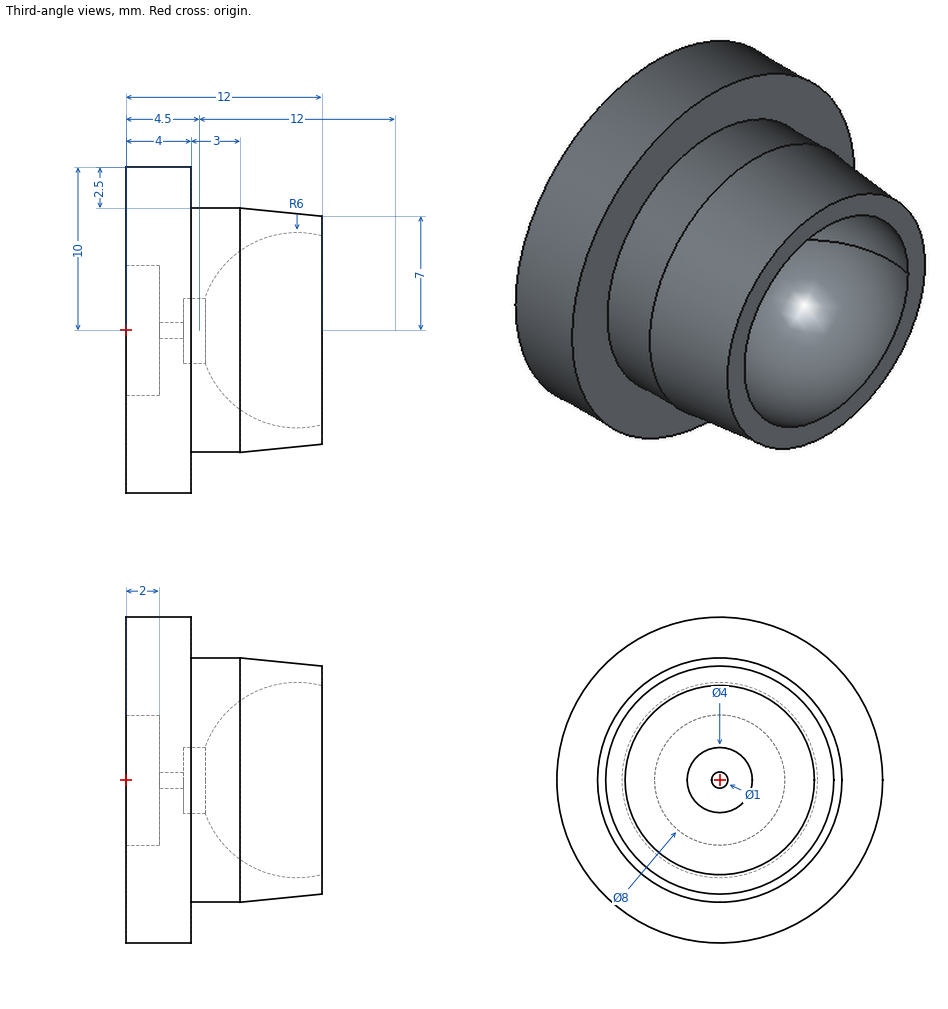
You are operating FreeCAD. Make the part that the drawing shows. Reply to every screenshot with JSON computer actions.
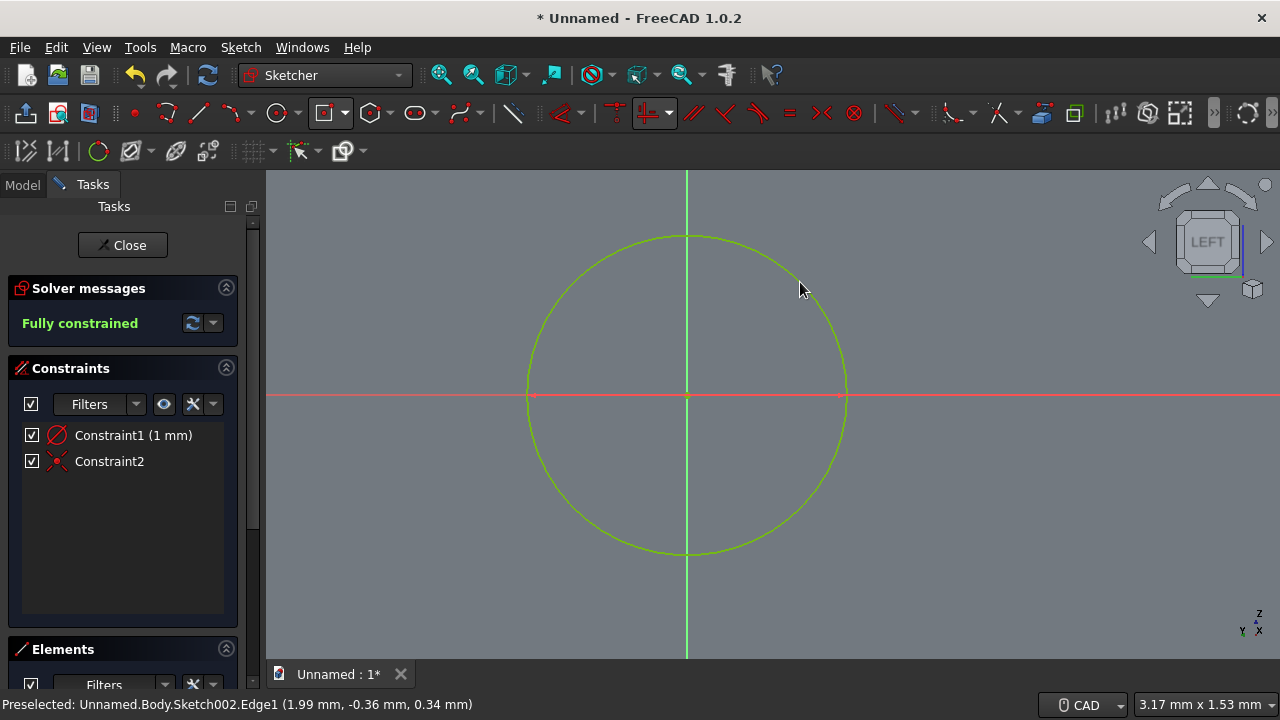
{"action": "left_click", "coordinate": [123, 245]}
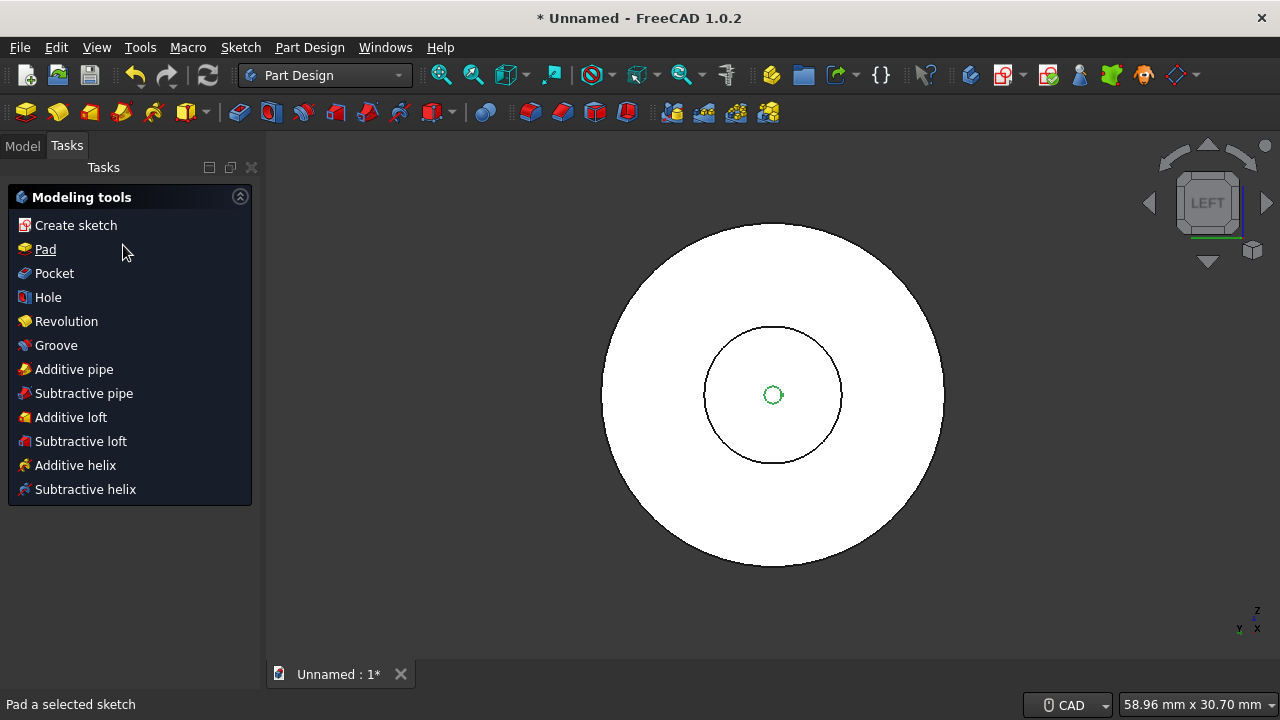
{"action": "left_click", "coordinate": [240, 112]}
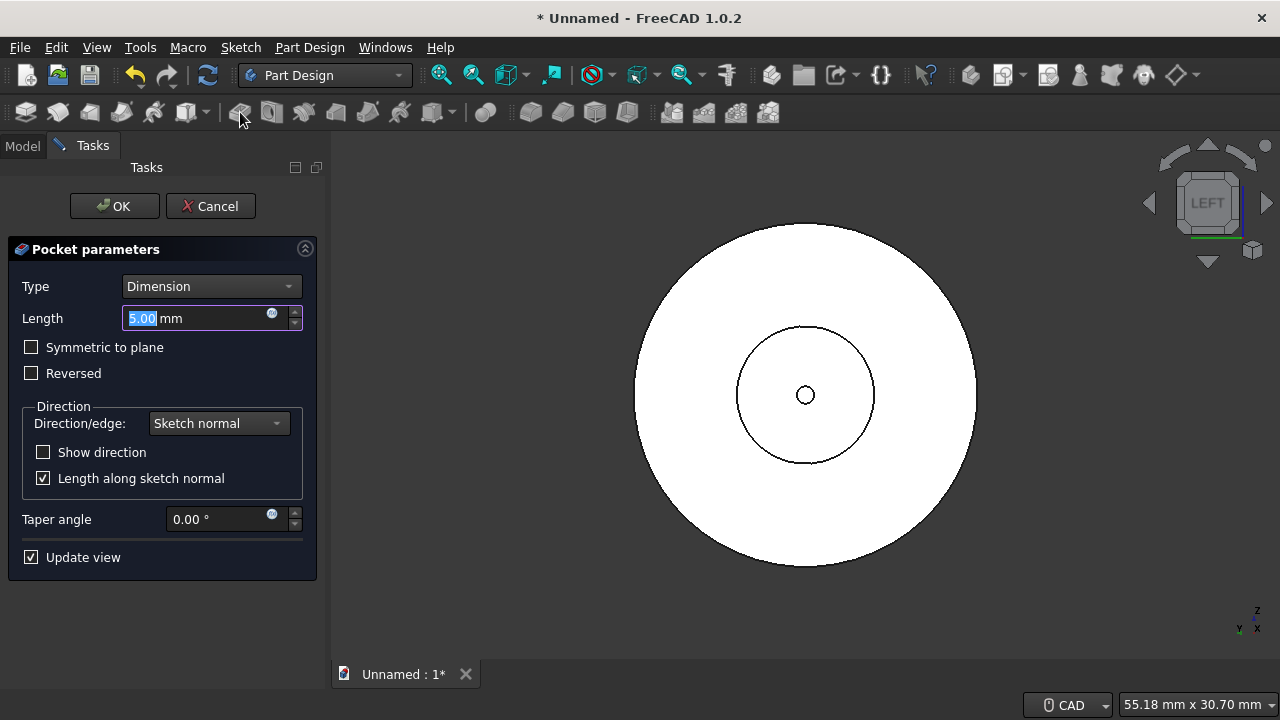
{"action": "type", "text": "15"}
{"action": "key", "text": "Tab"}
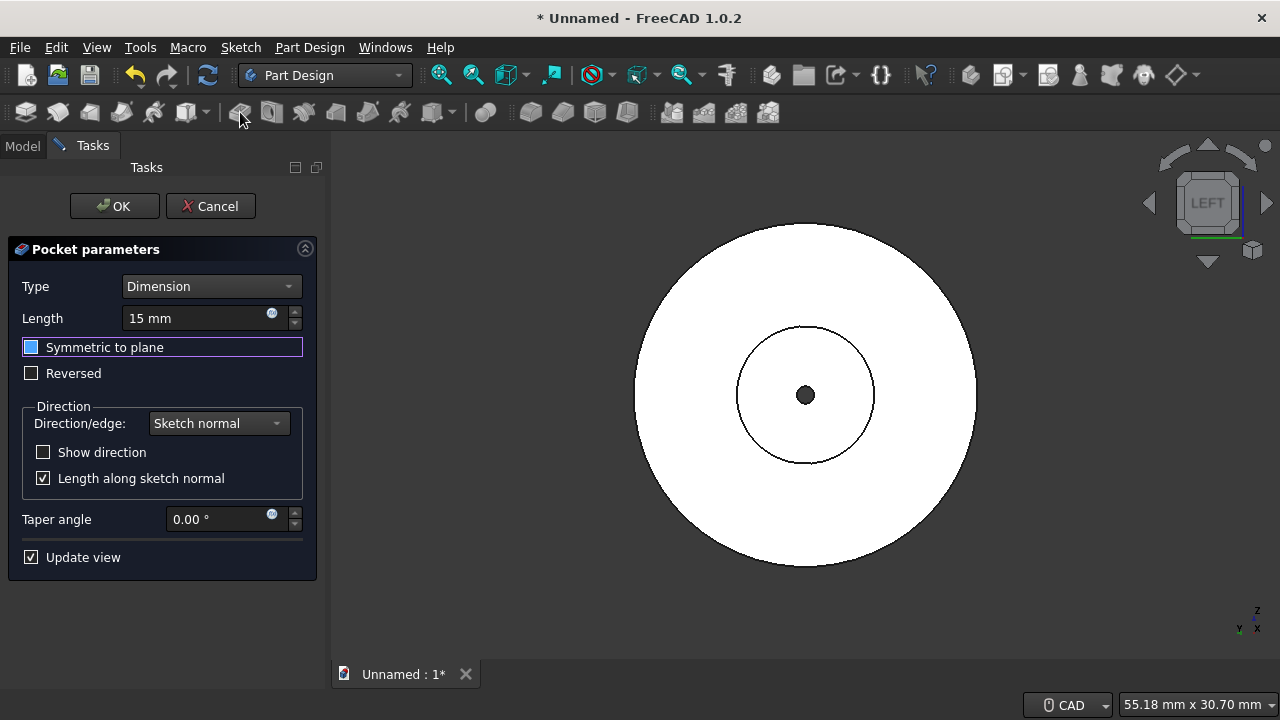
{"action": "left_click", "coordinate": [115, 206]}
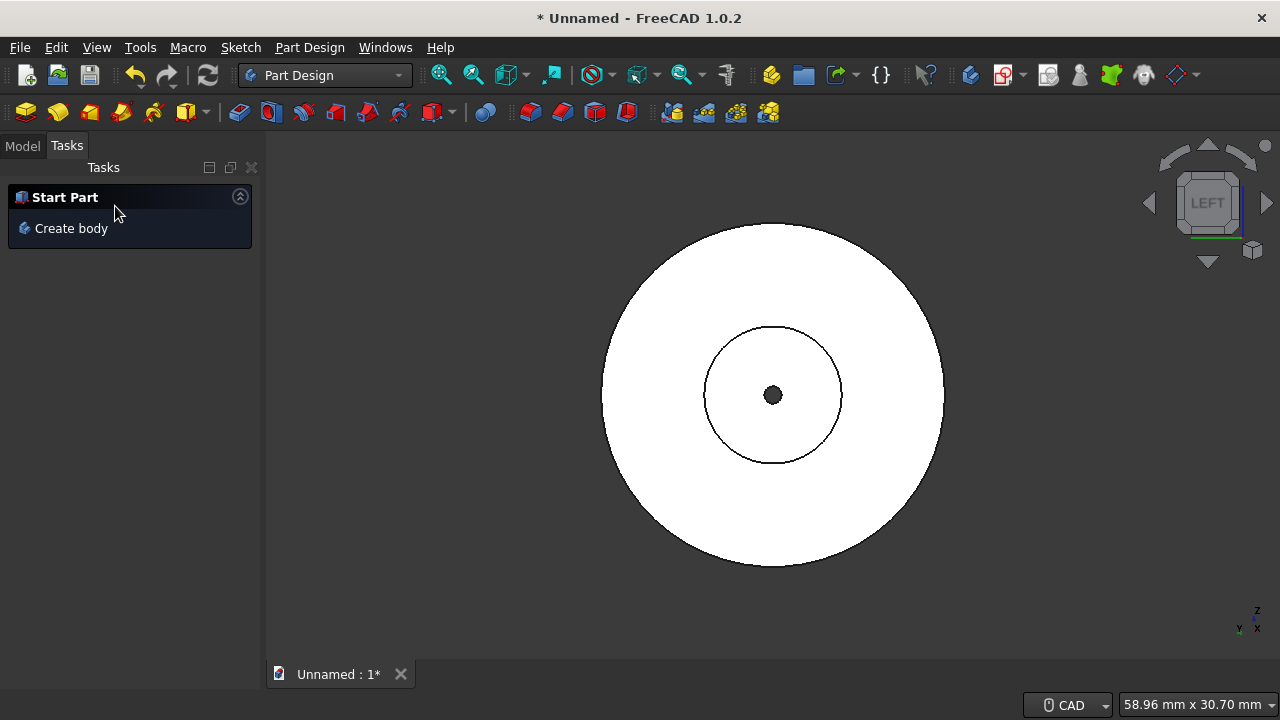
{"action": "left_click", "coordinate": [23, 145]}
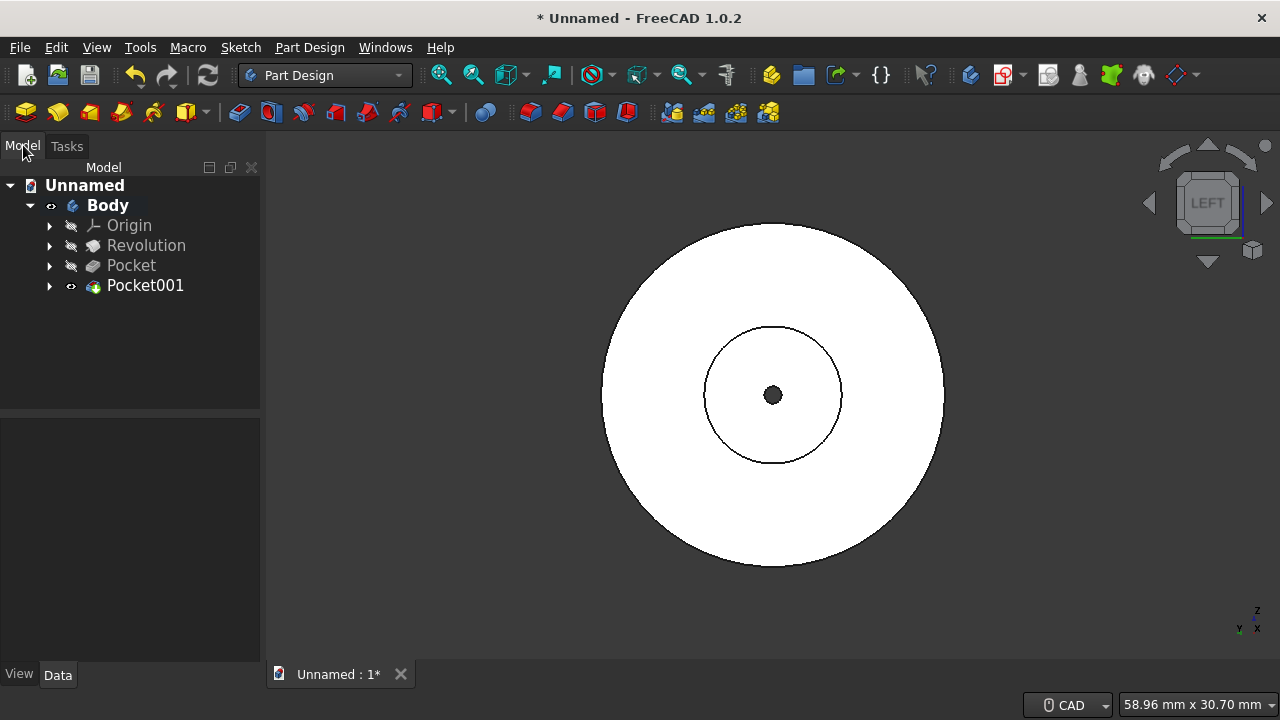
{"action": "left_click", "coordinate": [50, 226]}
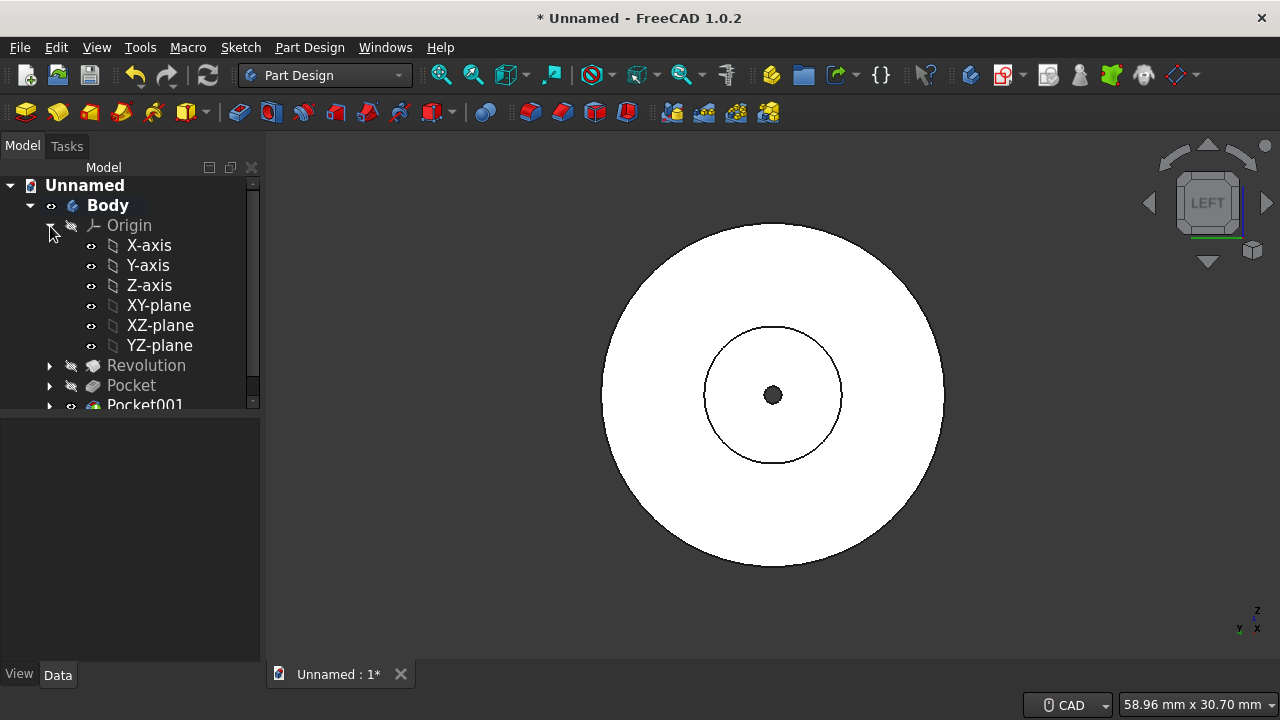
{"action": "left_click", "coordinate": [136, 346]}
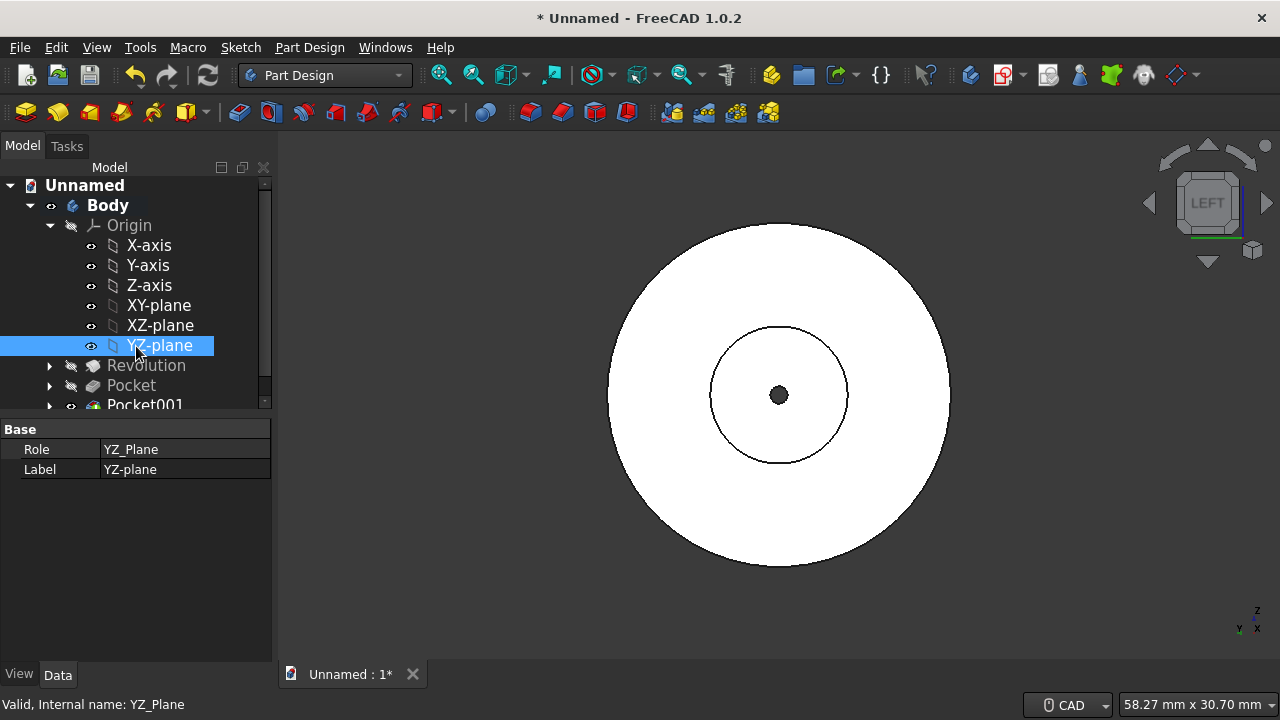
{"action": "left_click", "coordinate": [1176, 76]}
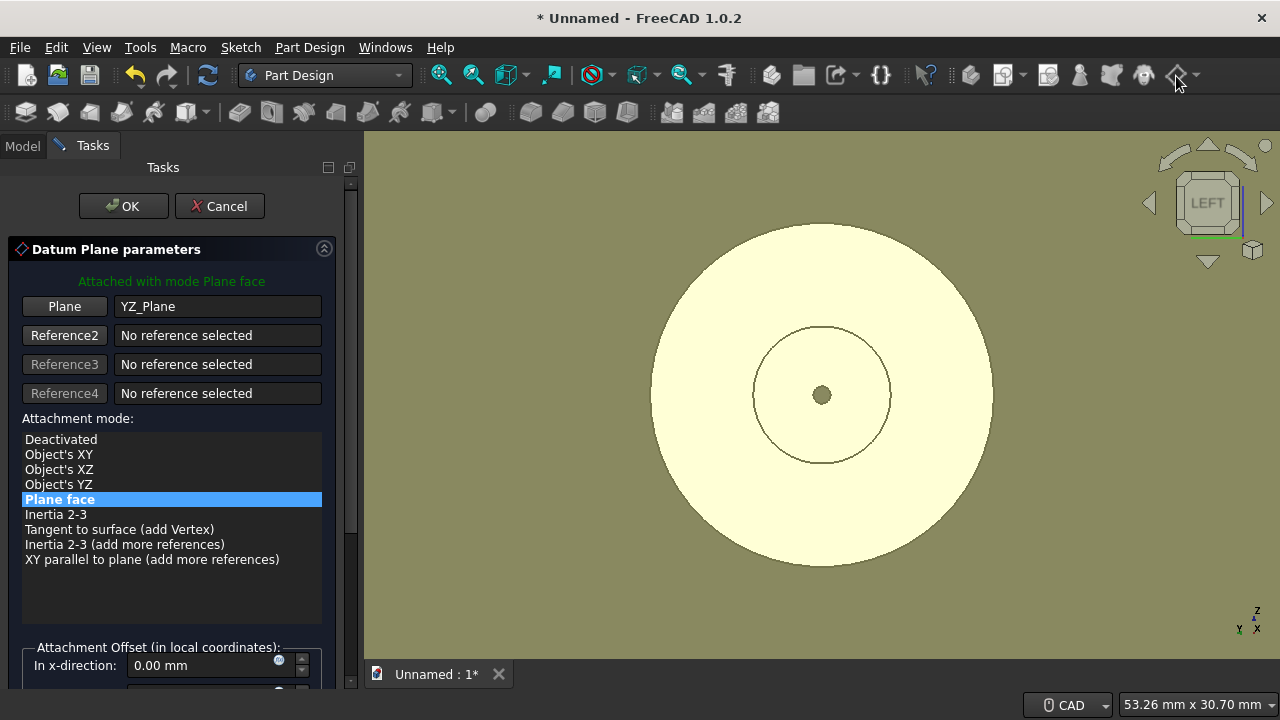
{"action": "scroll", "coordinate": [351, 432], "scroll_direction": "down", "scroll_amount": 2}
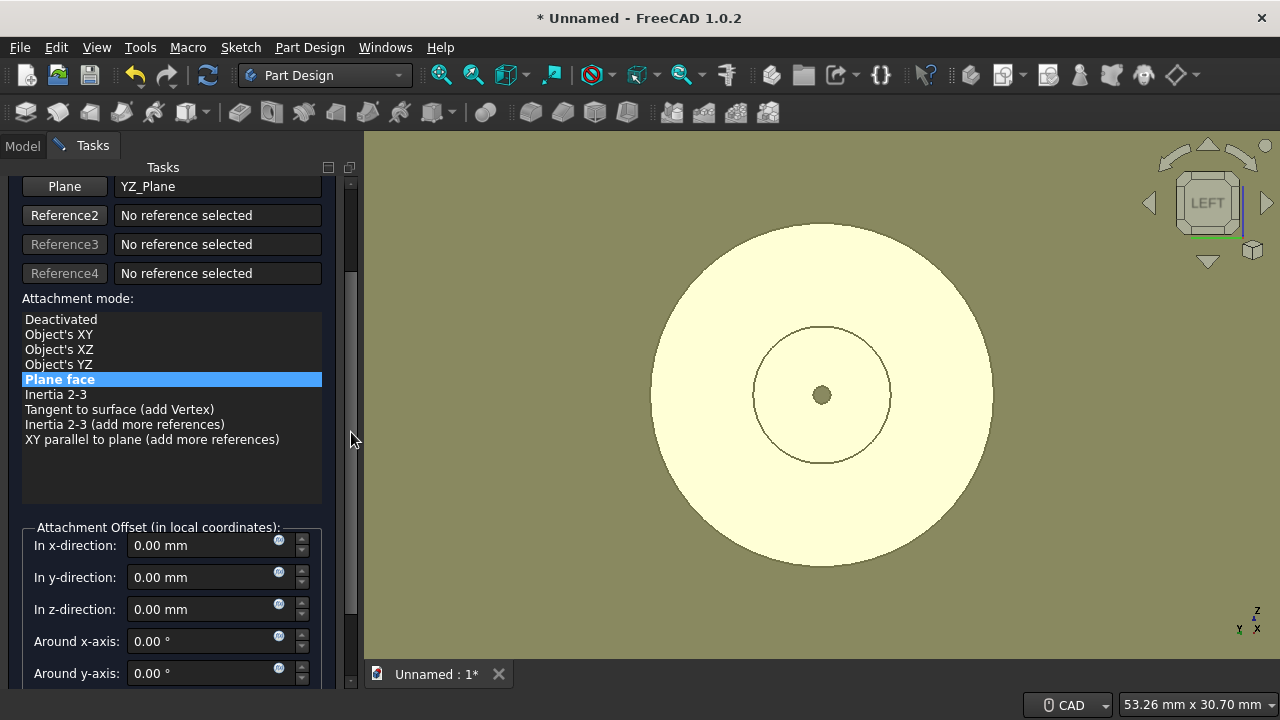
{"action": "triple_click", "coordinate": [210, 609]}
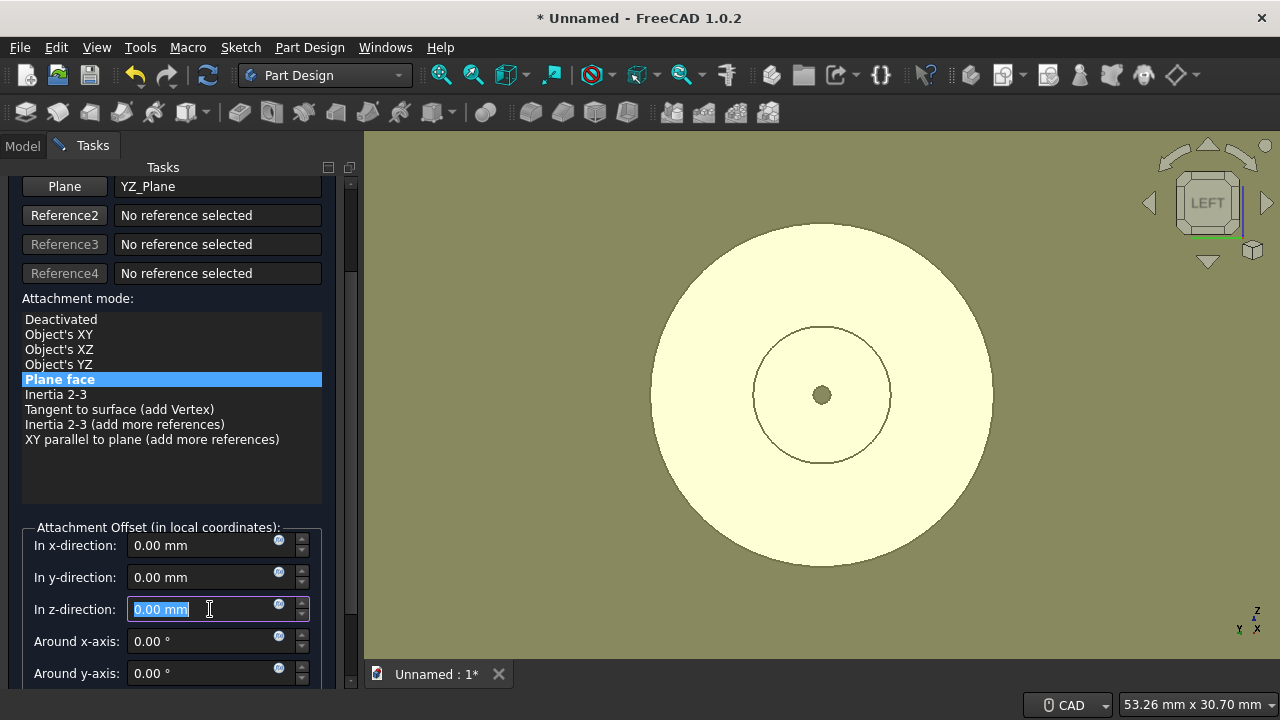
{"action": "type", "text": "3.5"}
{"action": "key", "text": "Tab"}